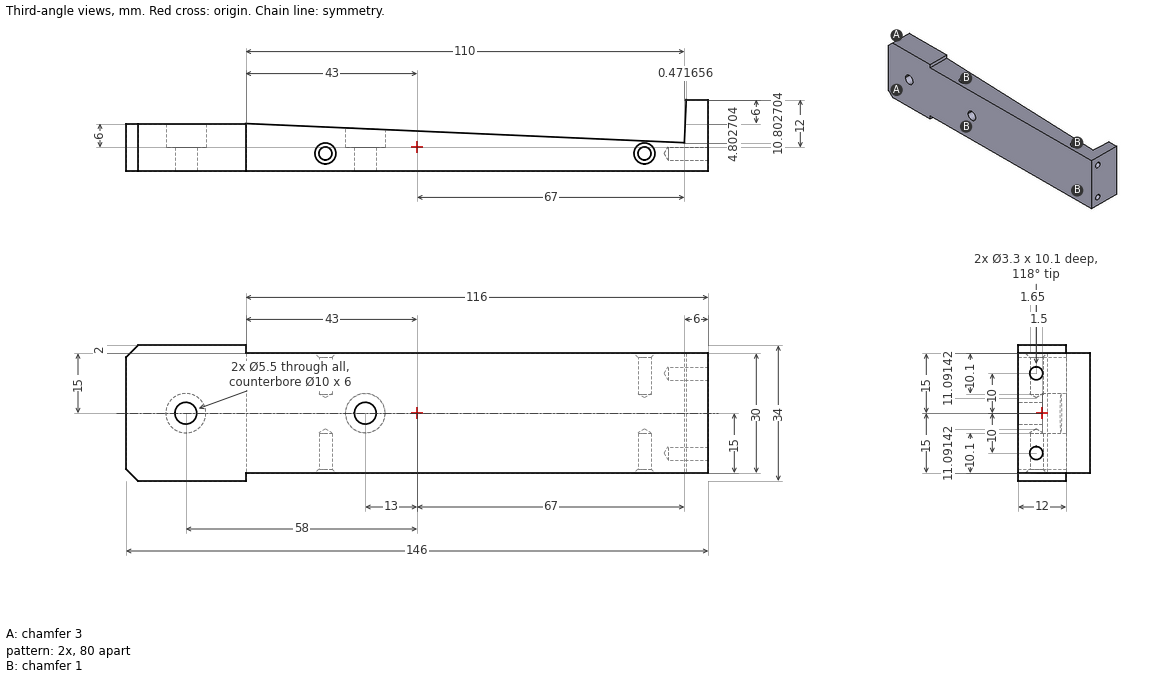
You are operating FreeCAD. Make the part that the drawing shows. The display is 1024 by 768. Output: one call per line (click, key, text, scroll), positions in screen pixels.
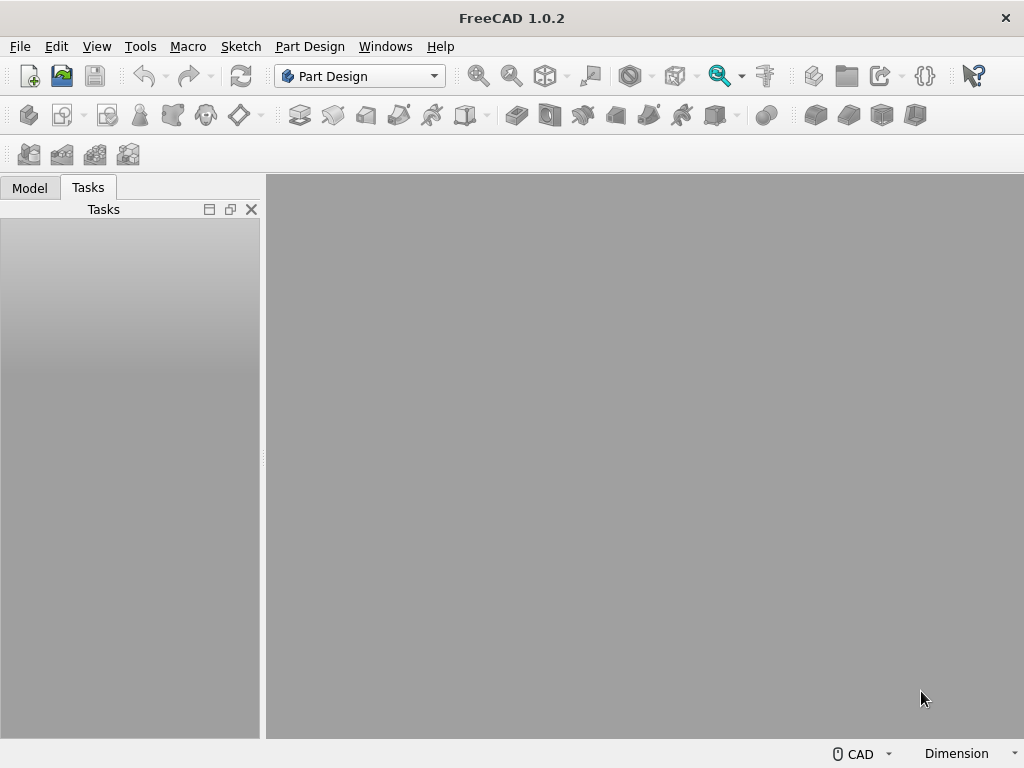
click(29, 76)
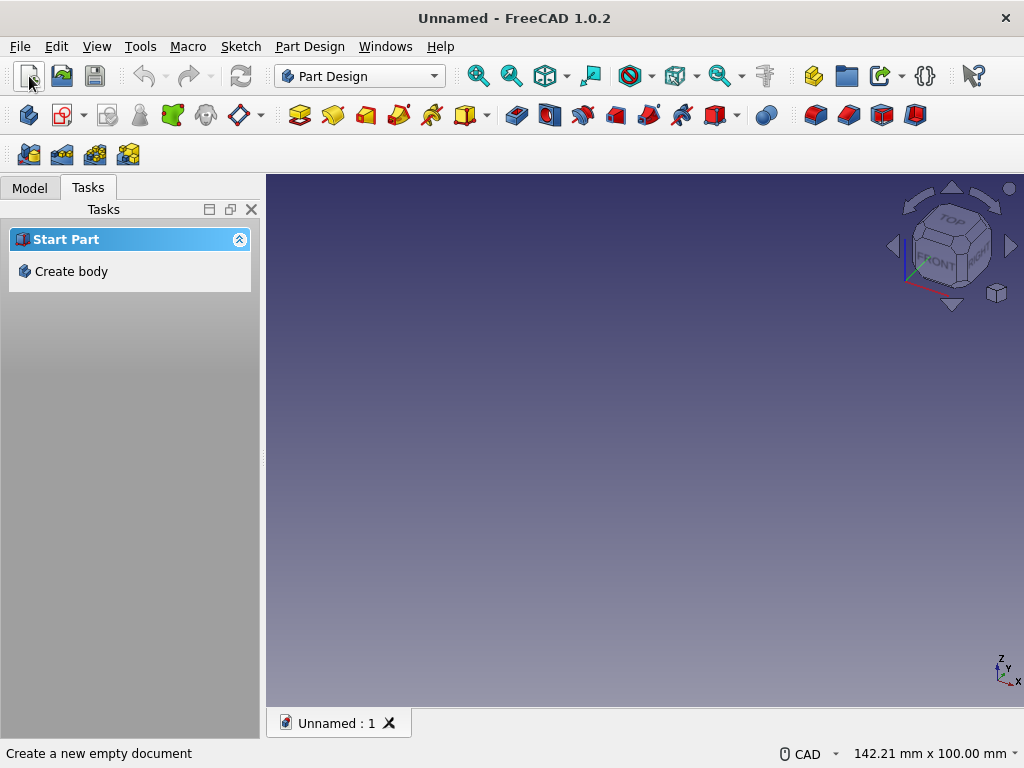
click(62, 116)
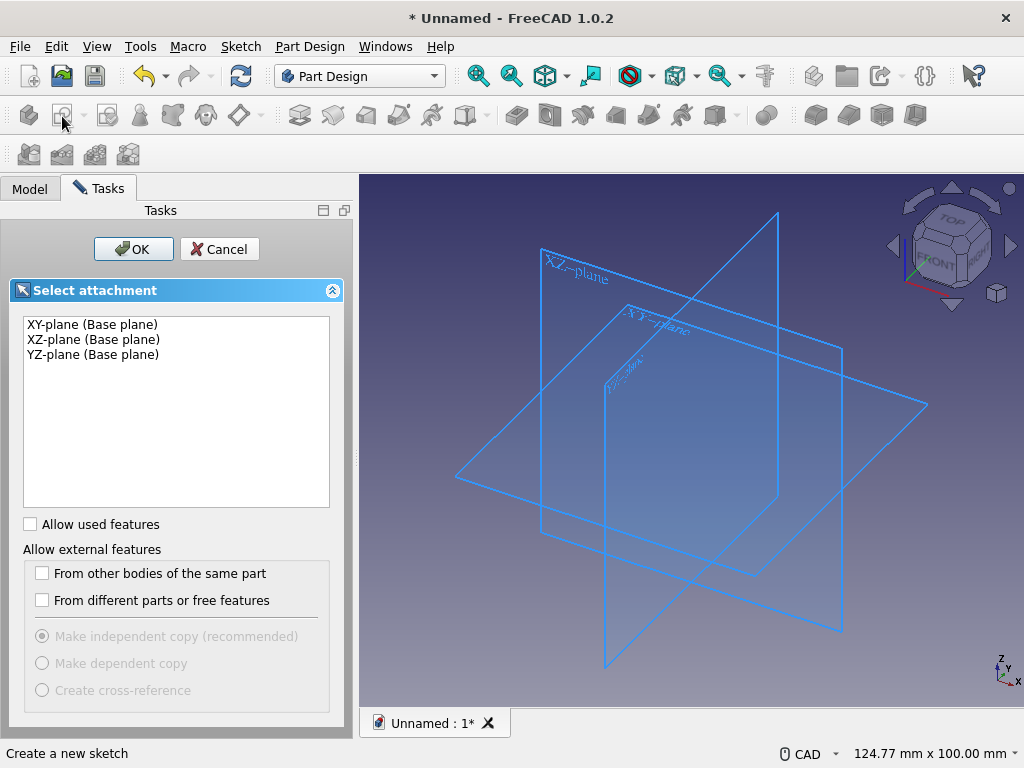
click(84, 340)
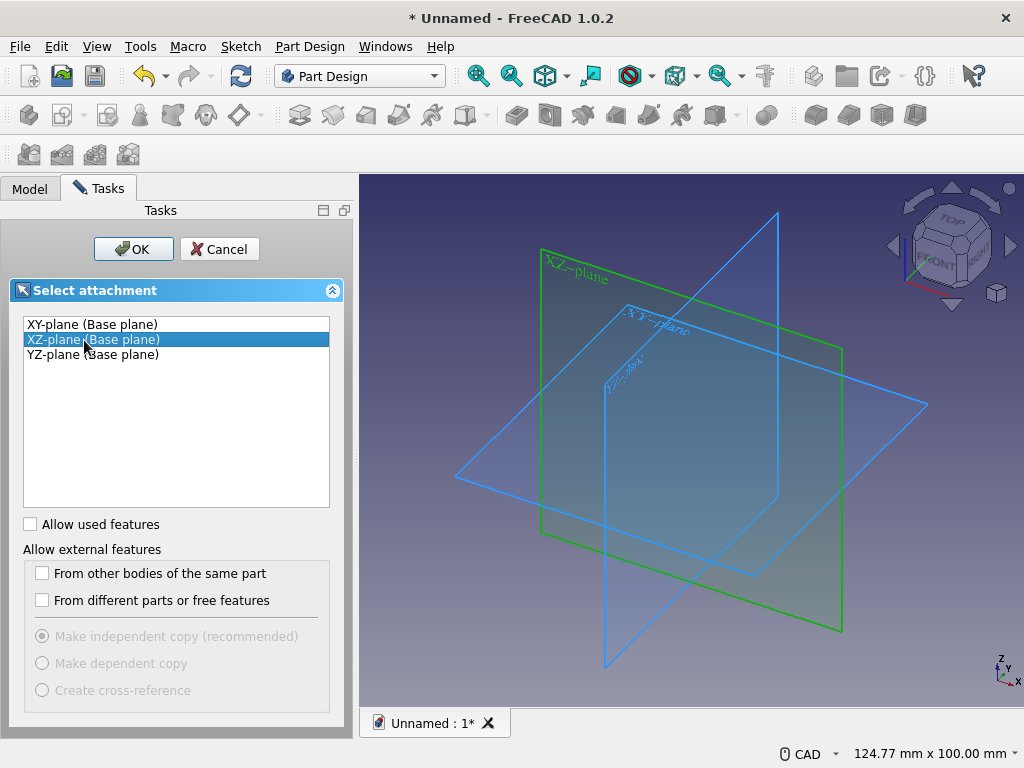
click(134, 249)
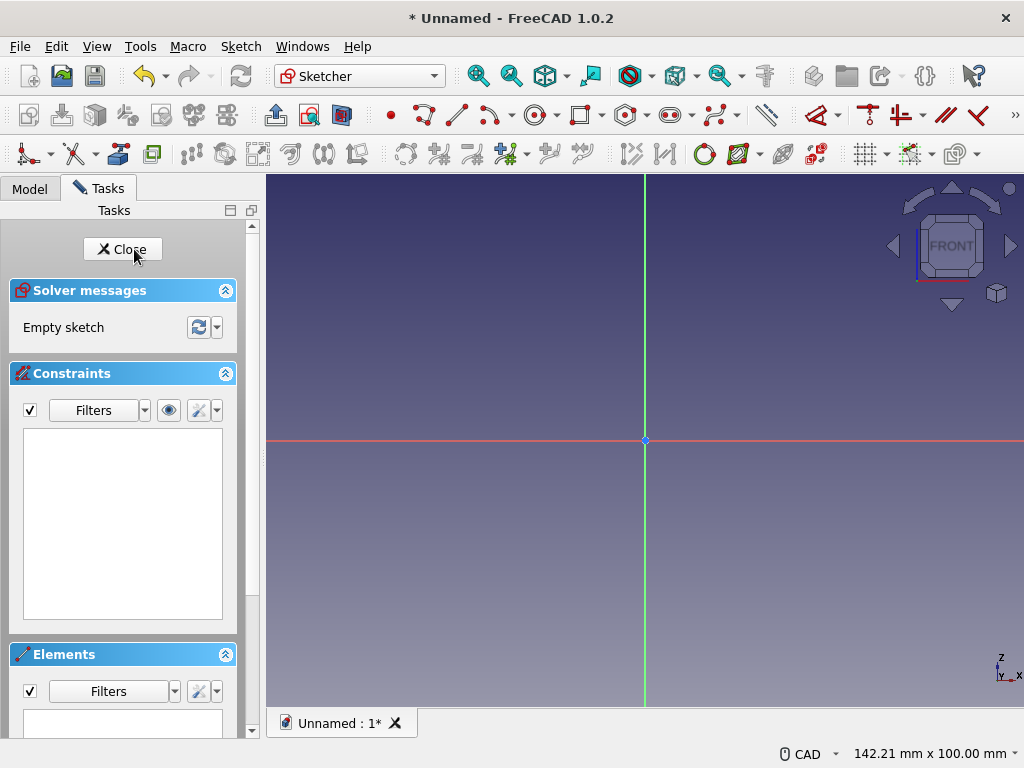
scroll(493, 440, down, 3)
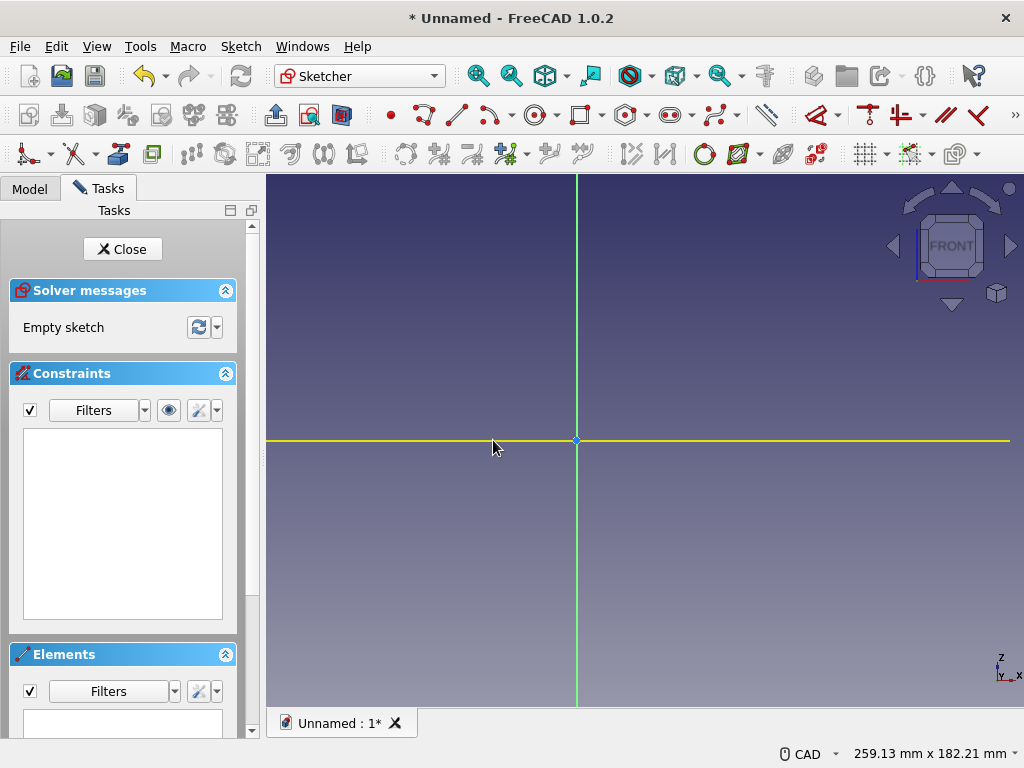
key(g)
key(v)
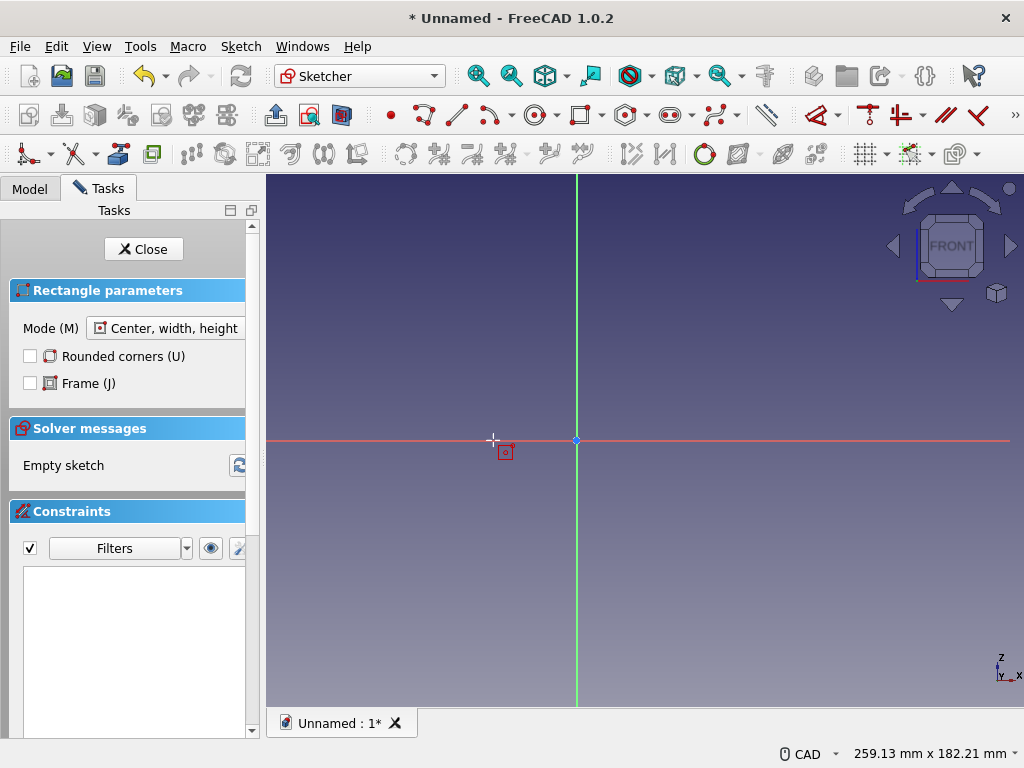
click(577, 440)
move(790, 391)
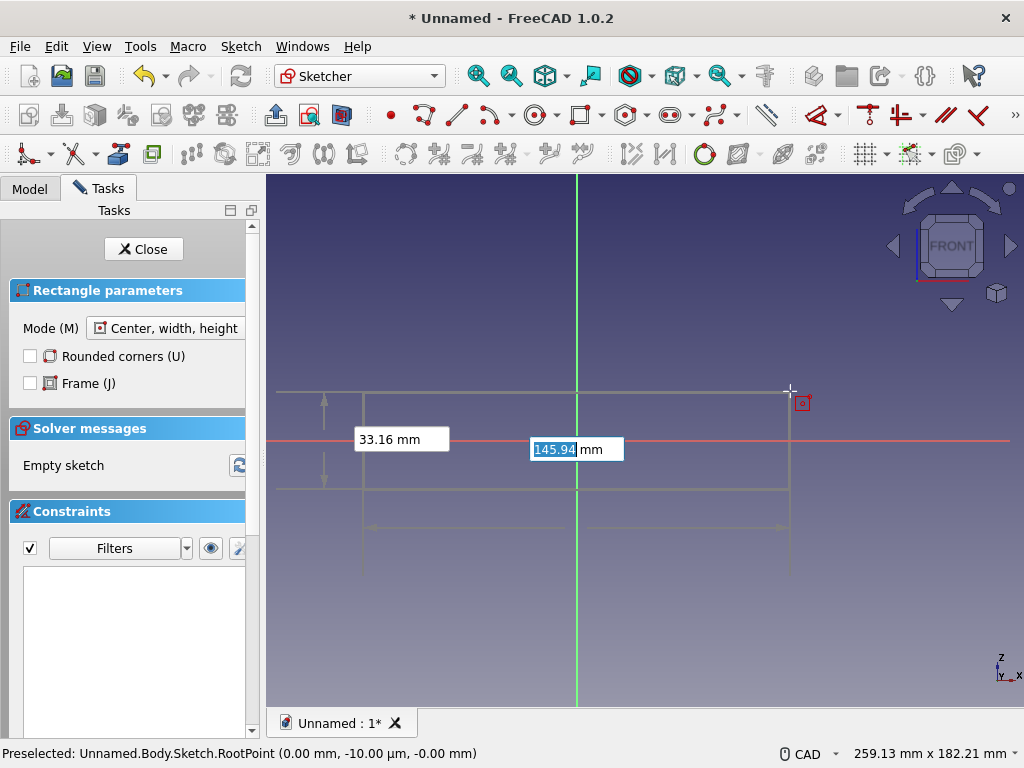
text(146)
key(Tab)
text(34)
key(Return)
key(Escape)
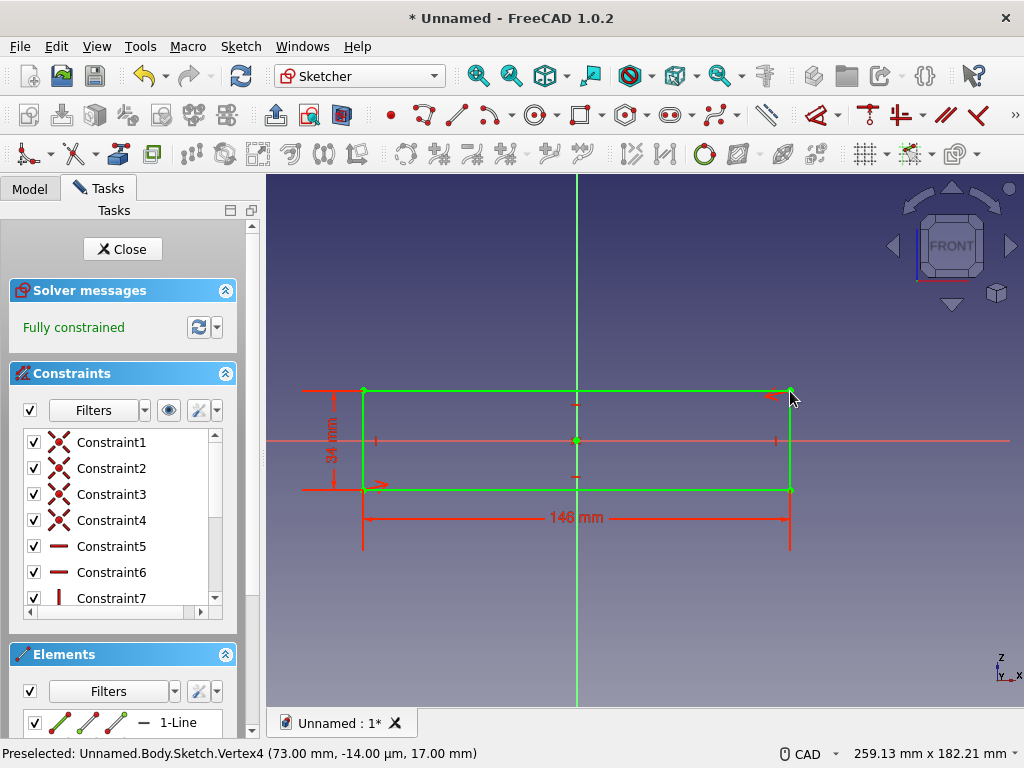
click(123, 249)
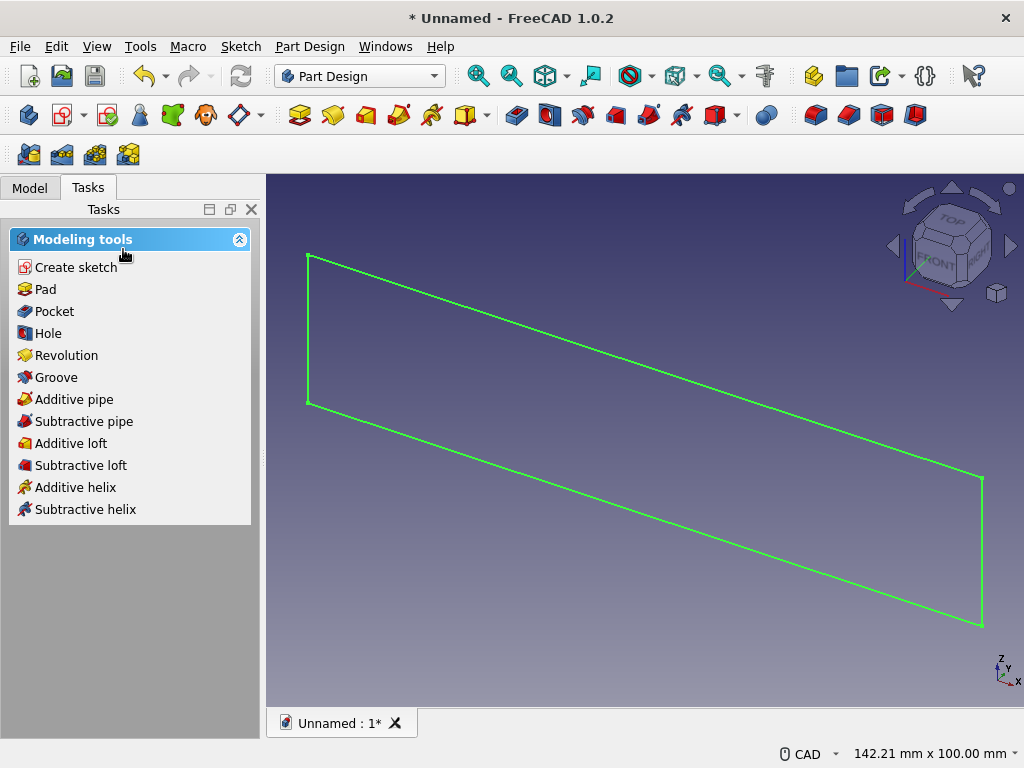
click(300, 116)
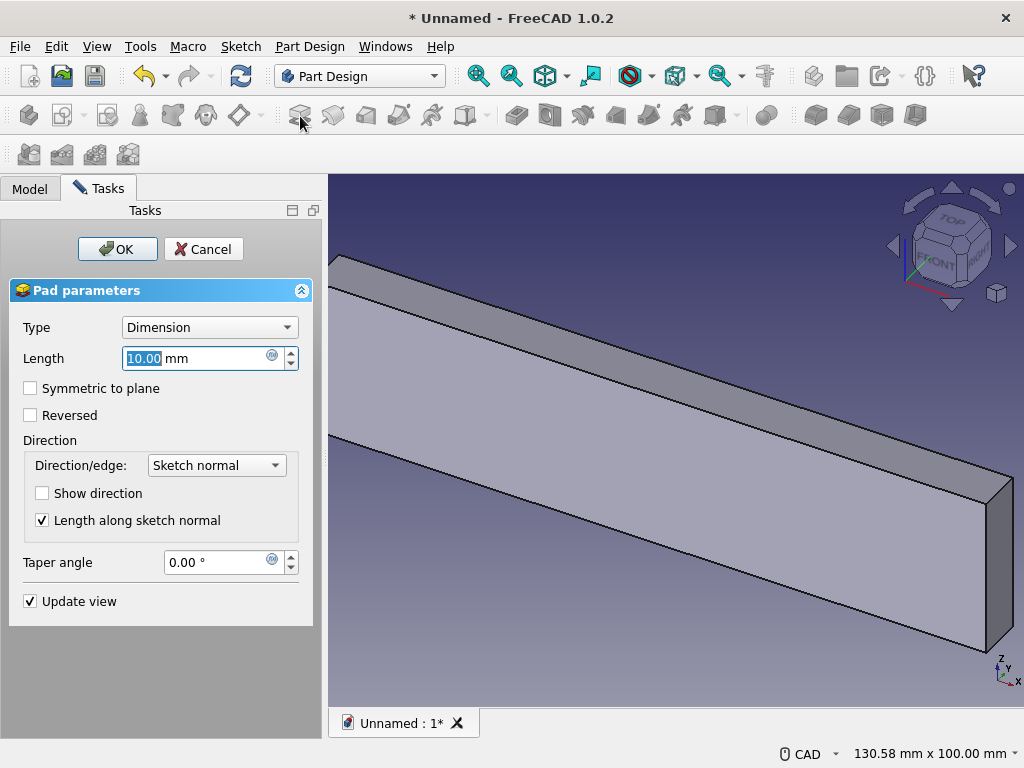
text(12)
key(Tab)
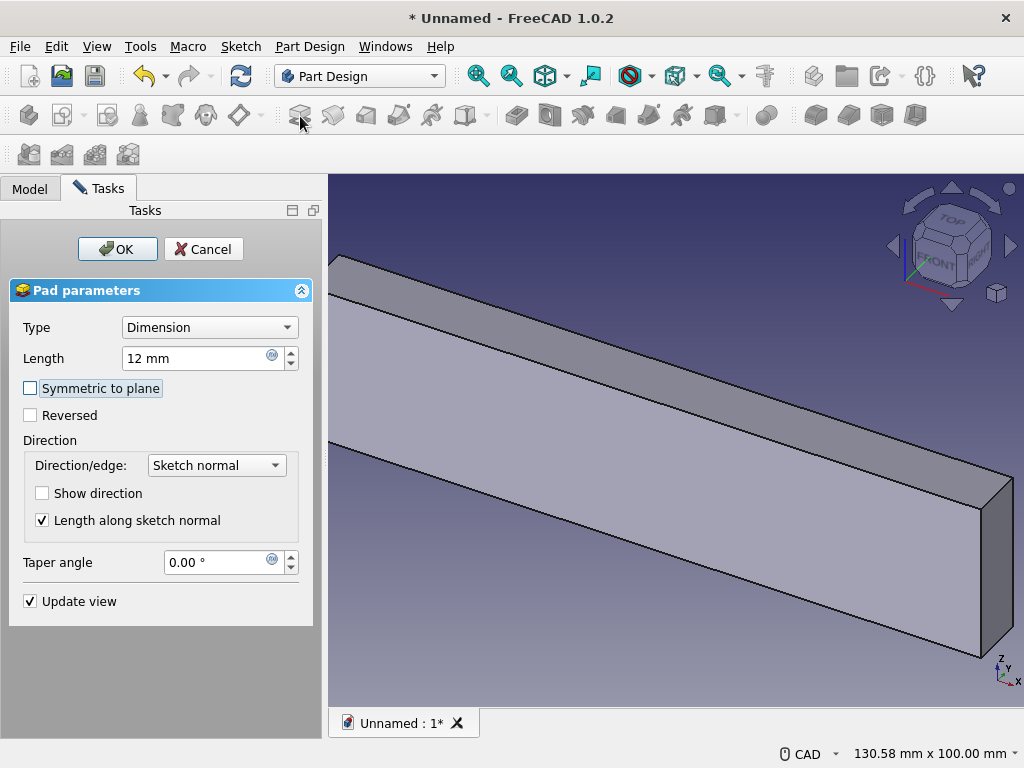
click(31, 388)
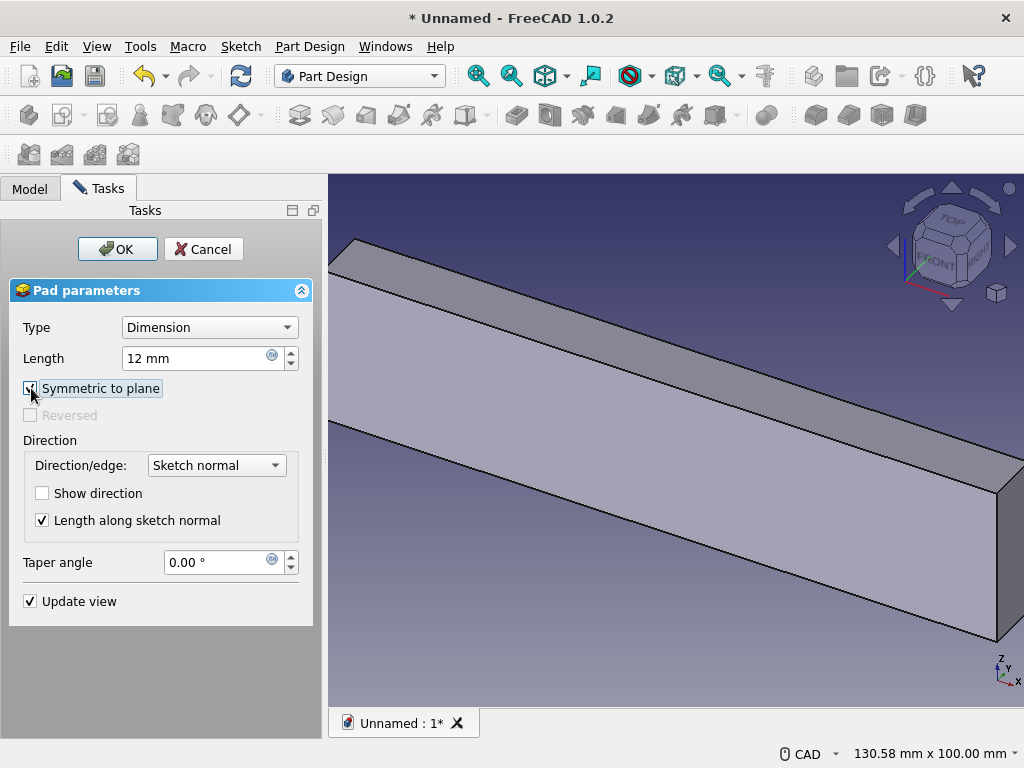
click(118, 249)